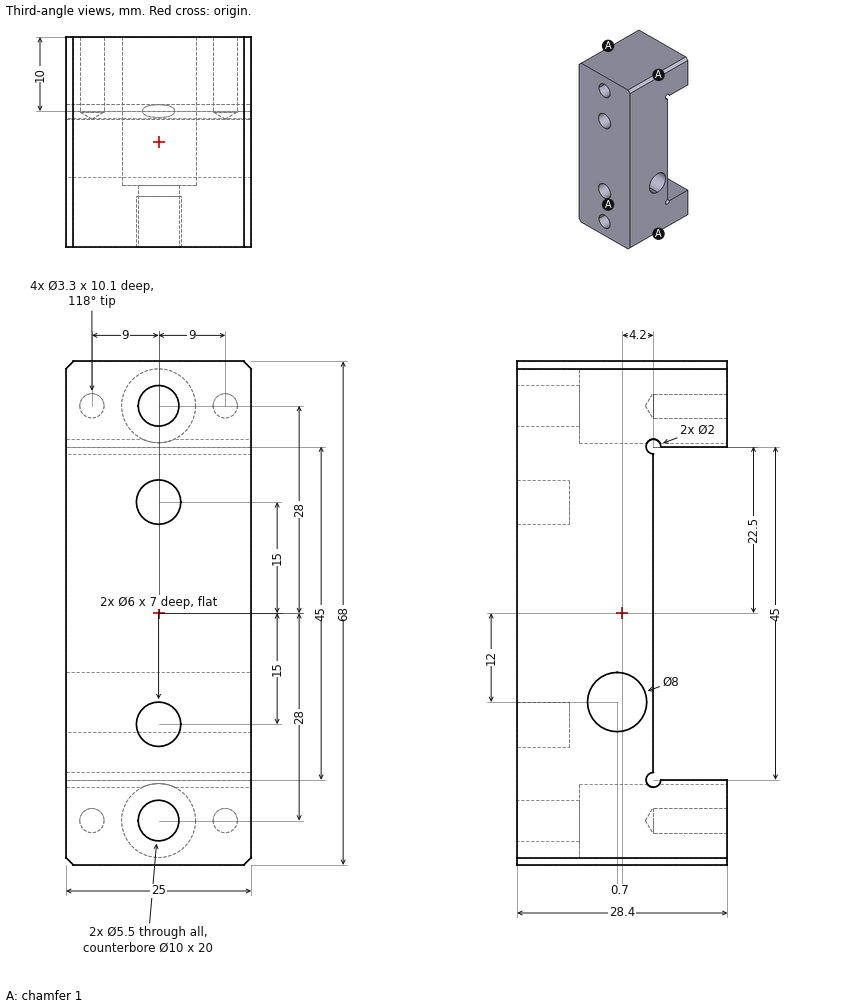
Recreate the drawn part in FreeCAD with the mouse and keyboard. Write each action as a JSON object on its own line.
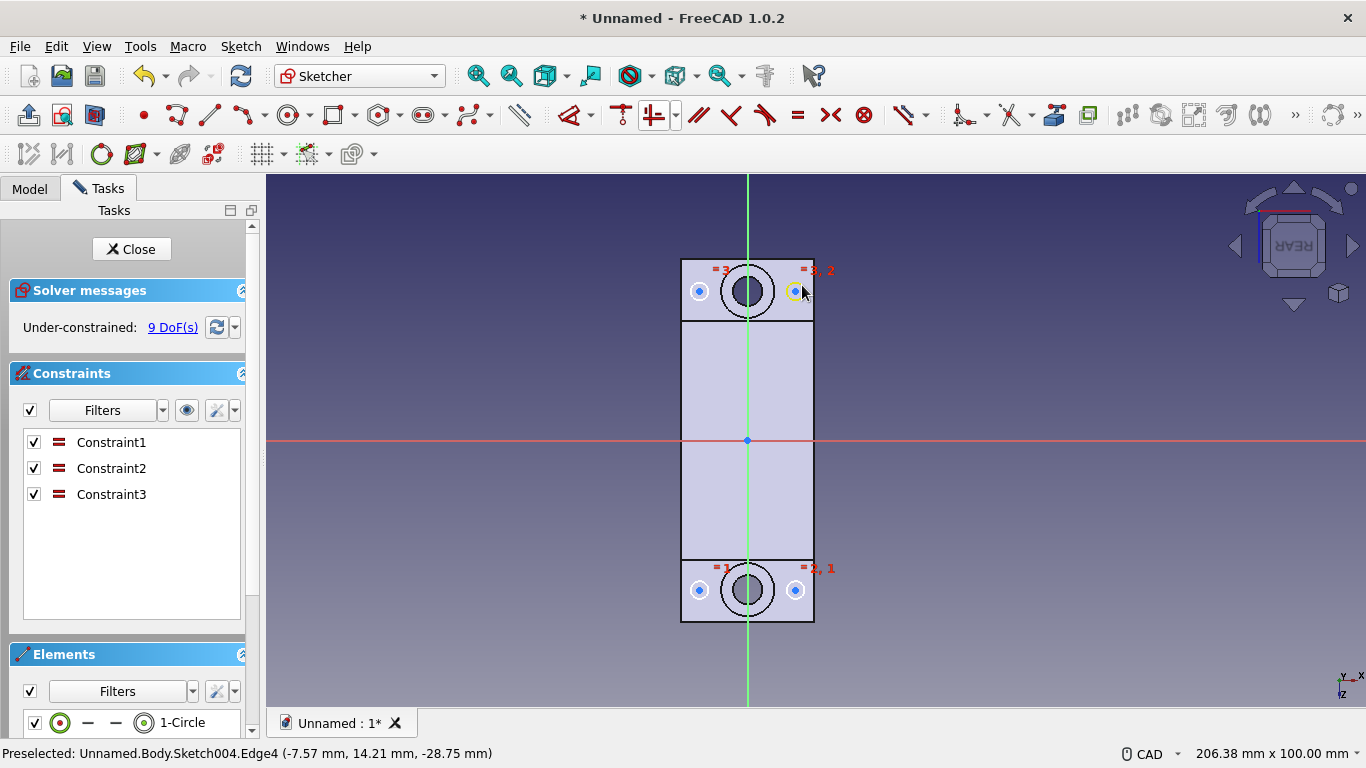
{"action": "left_click", "coordinate": [700, 590]}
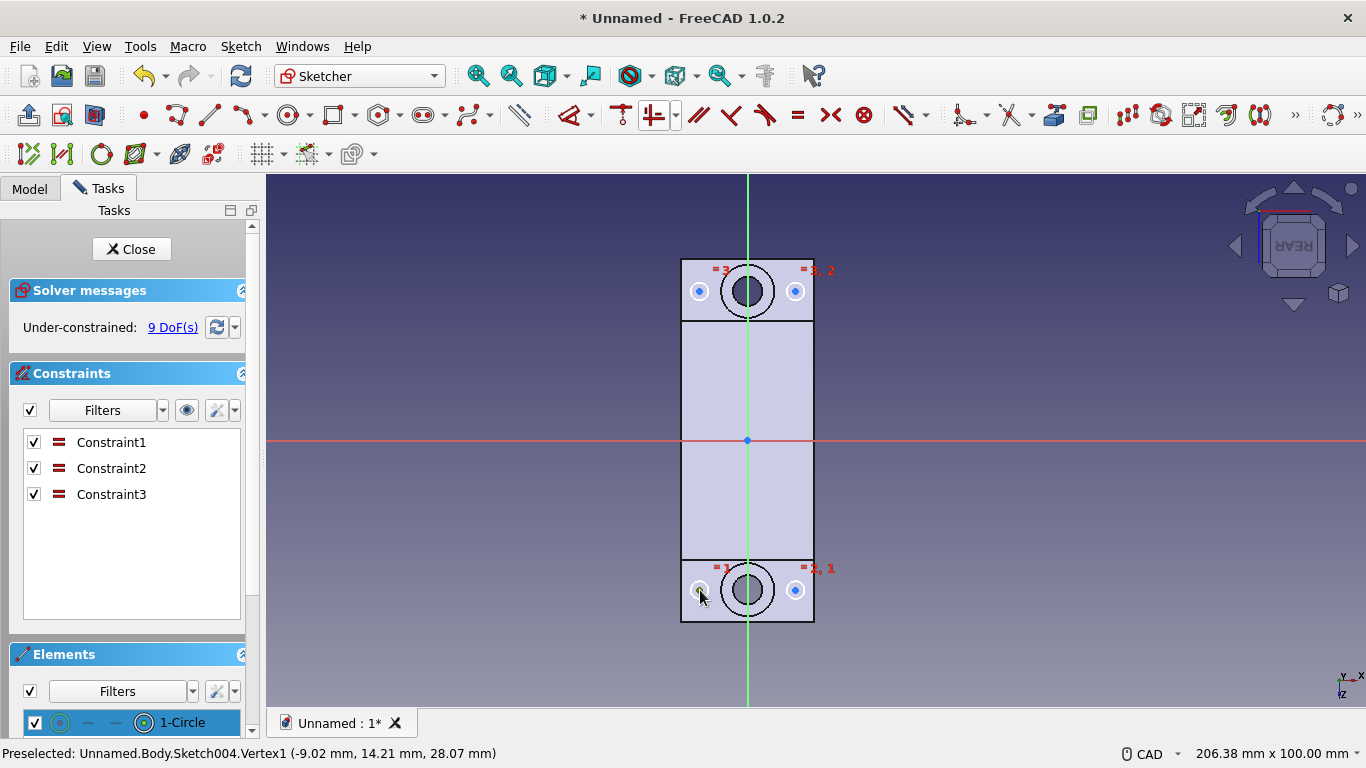
{"action": "left_click", "coordinate": [796, 590]}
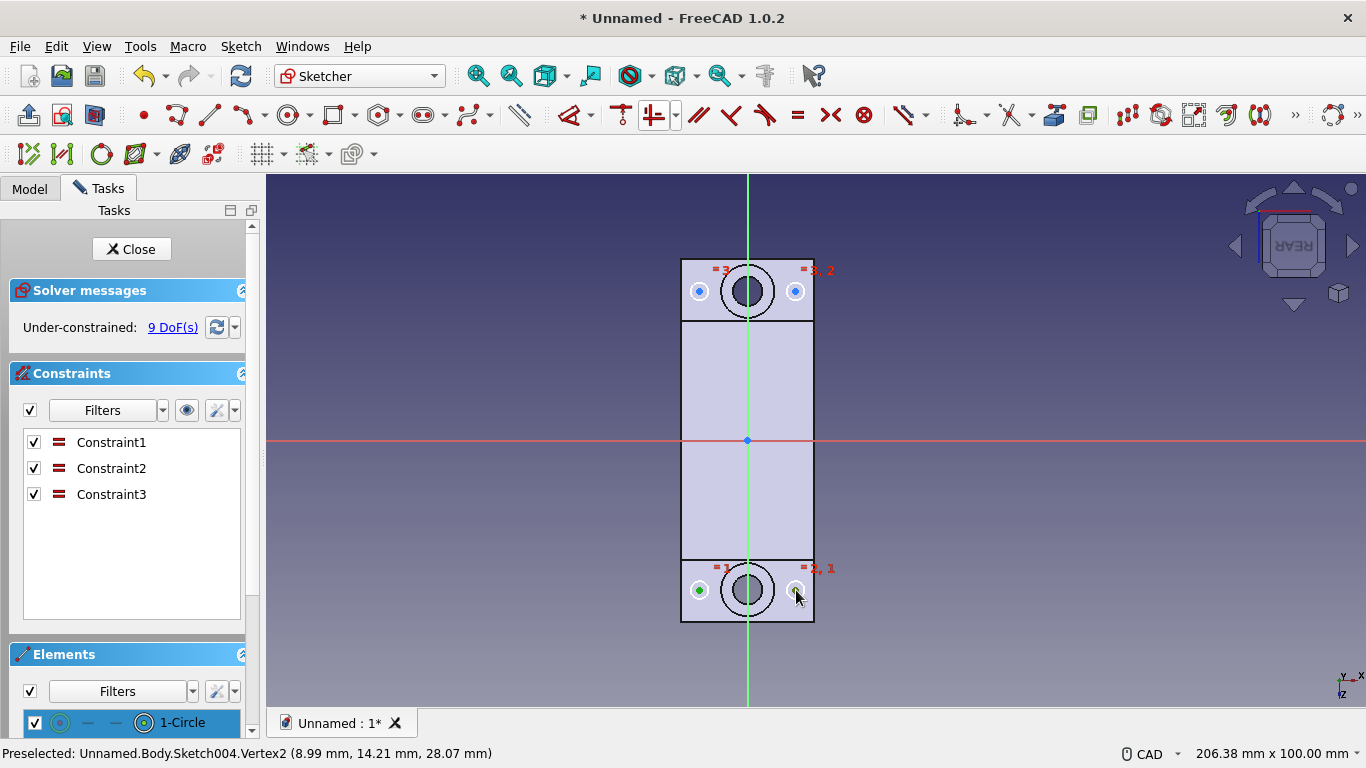
{"action": "key", "text": "h"}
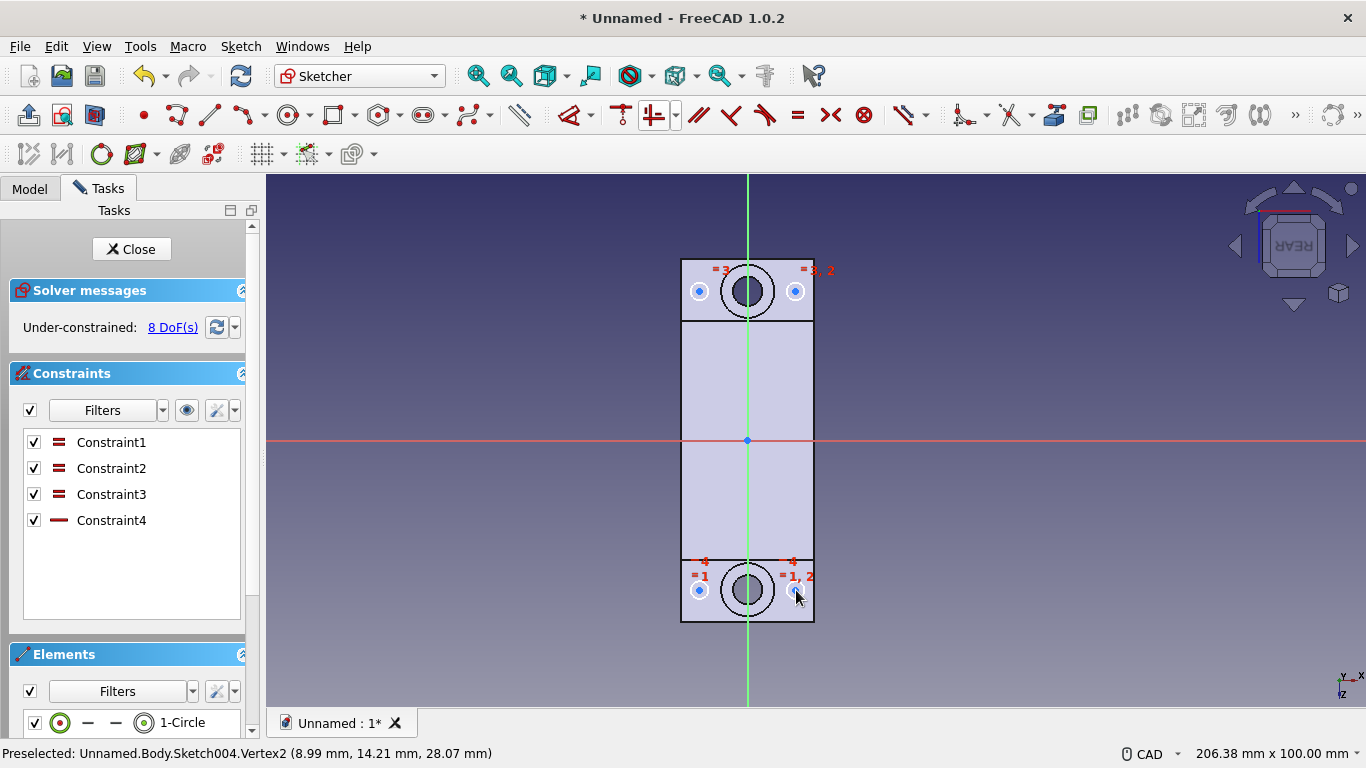
{"action": "left_click", "coordinate": [796, 590]}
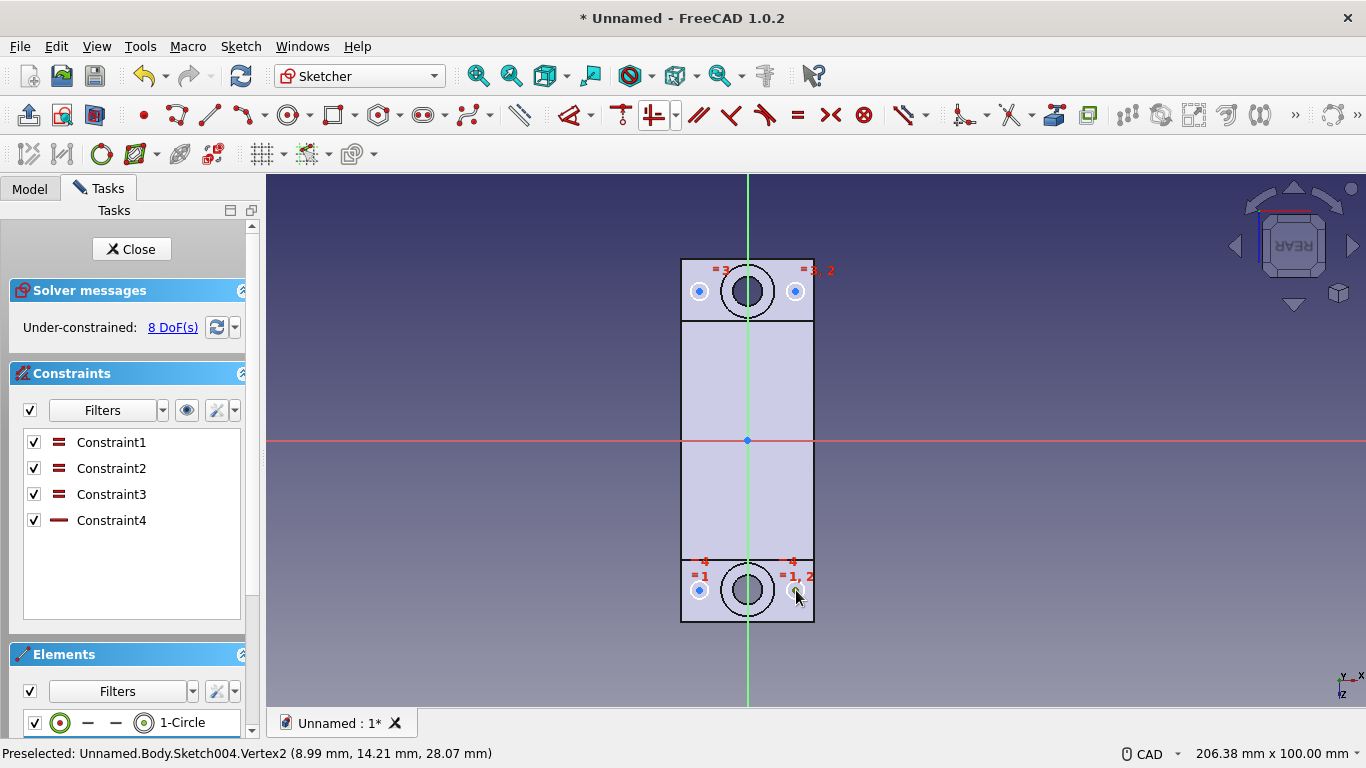
{"action": "left_click", "coordinate": [796, 292]}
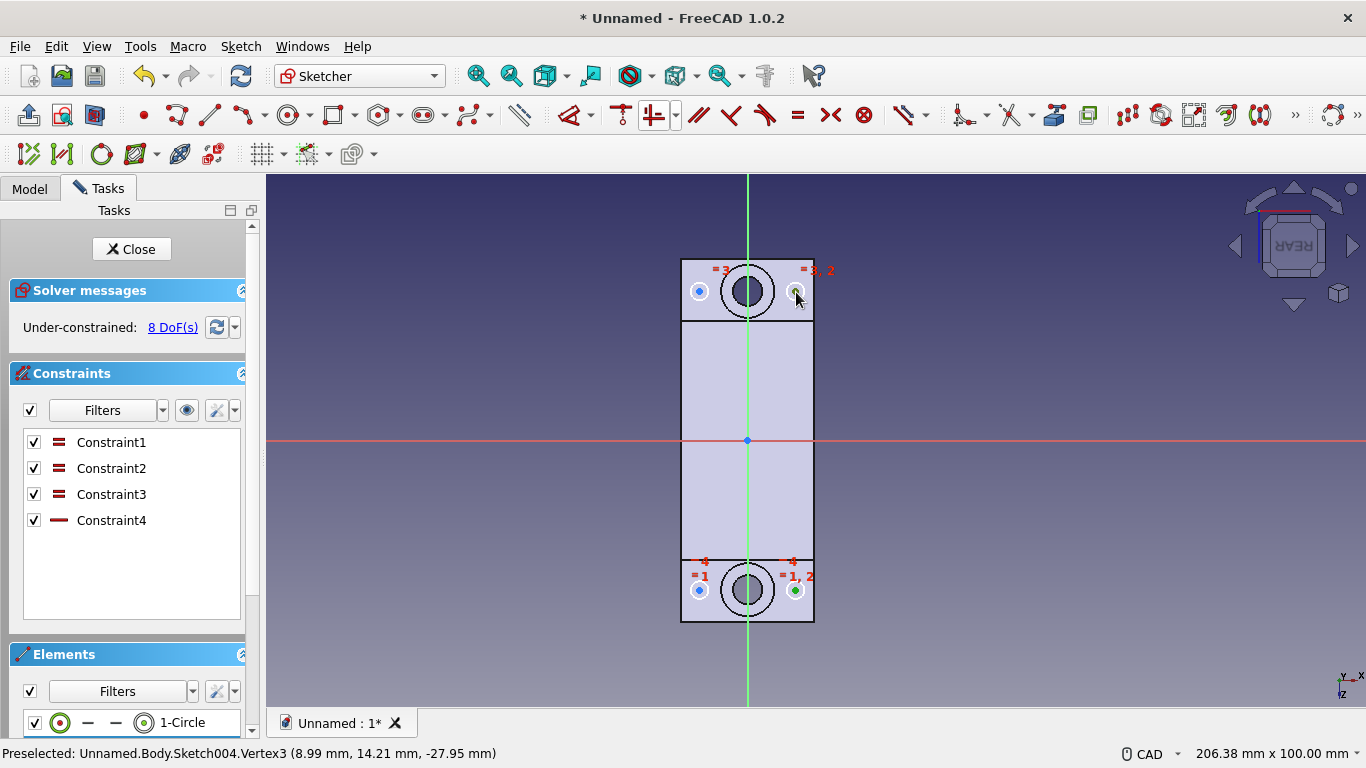
{"action": "key", "text": "v"}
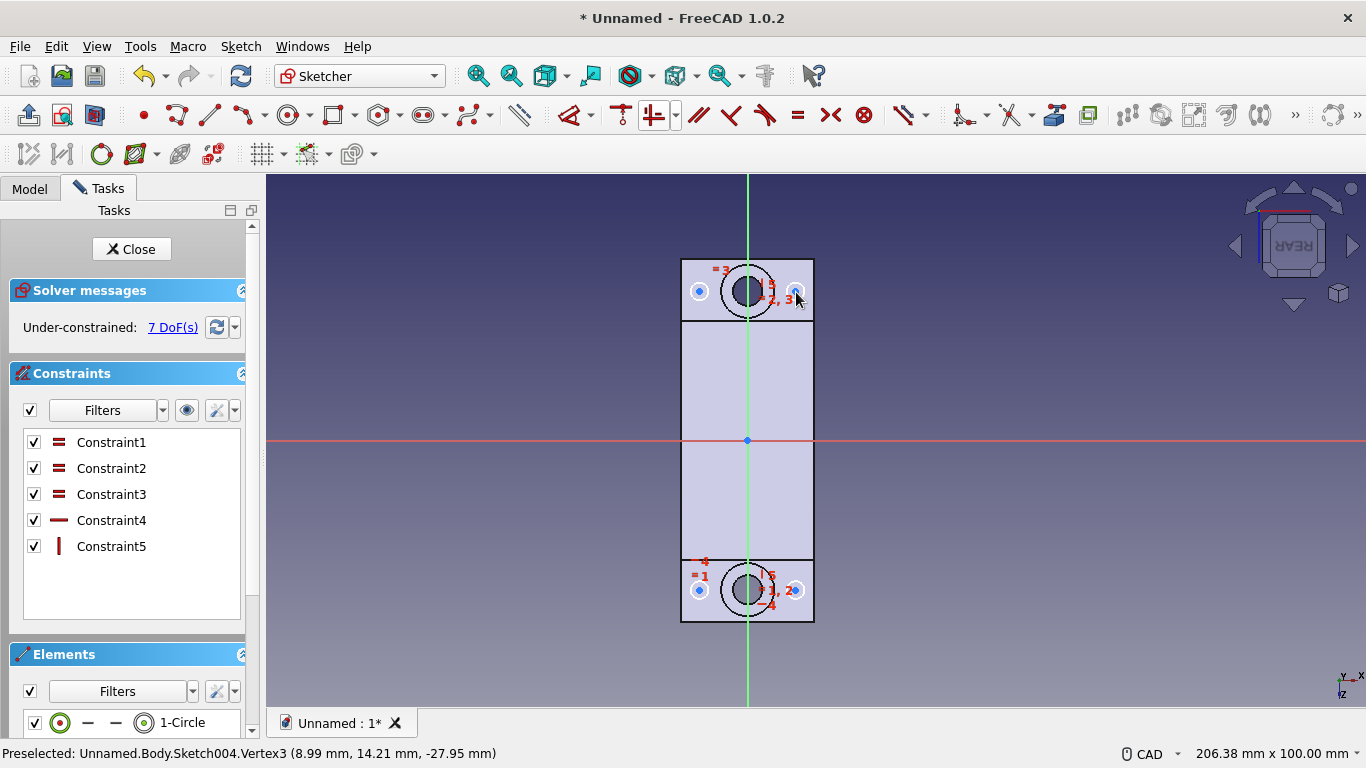
{"action": "left_click", "coordinate": [700, 590]}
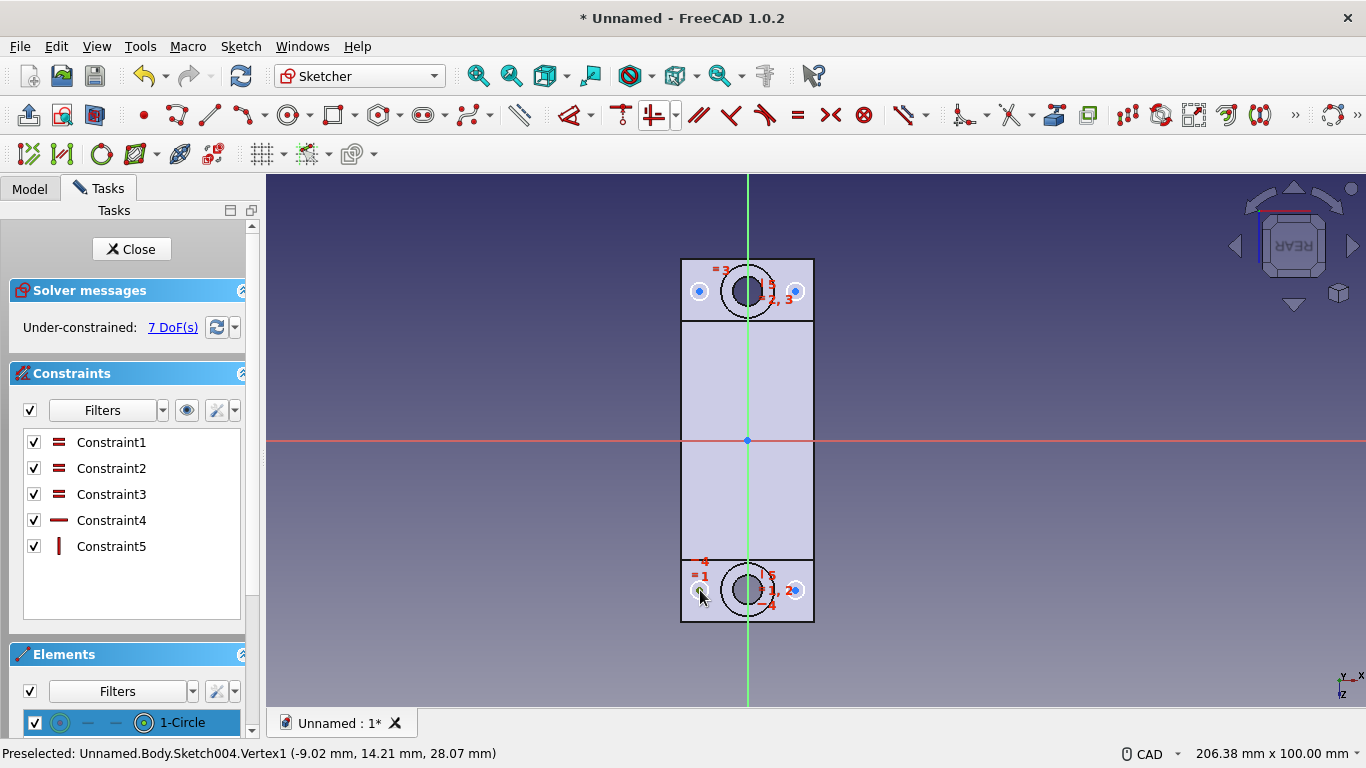
{"action": "left_click", "coordinate": [700, 292]}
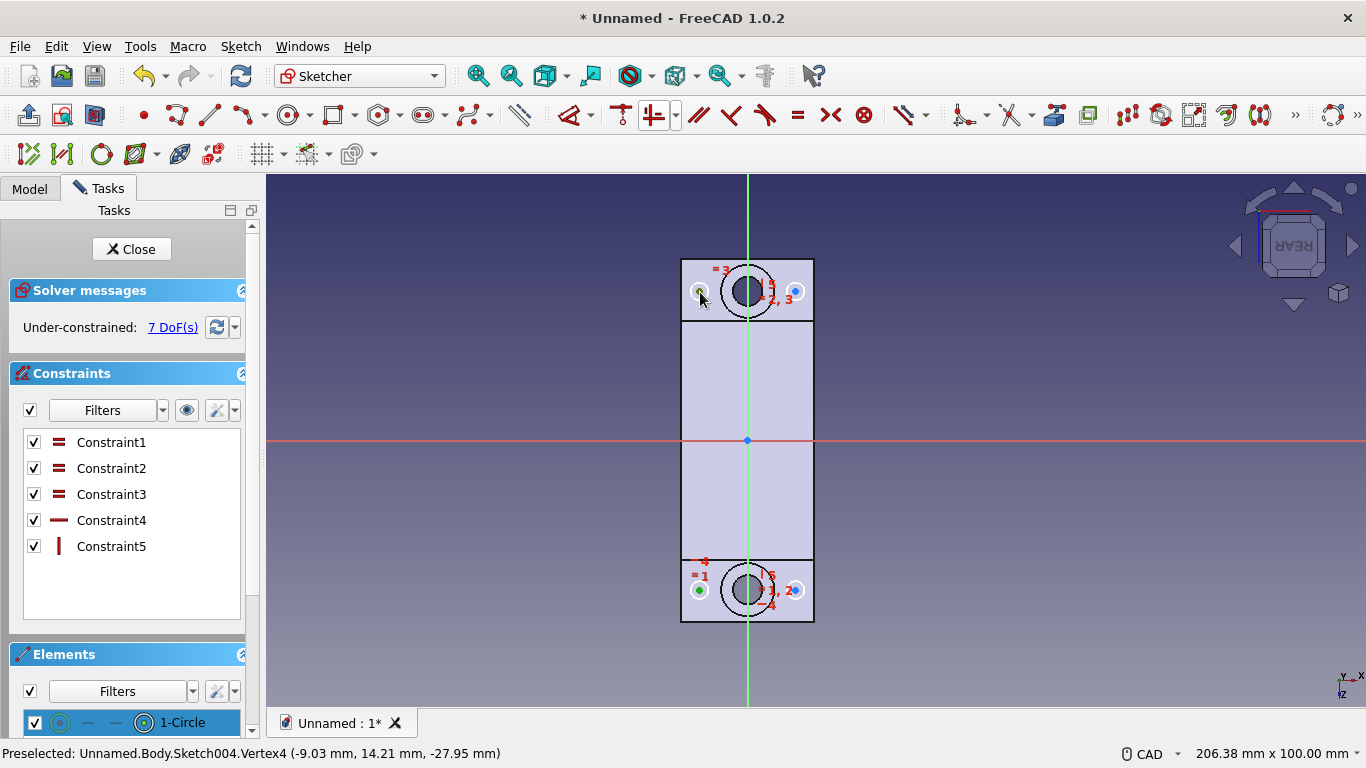
{"action": "key", "text": "v"}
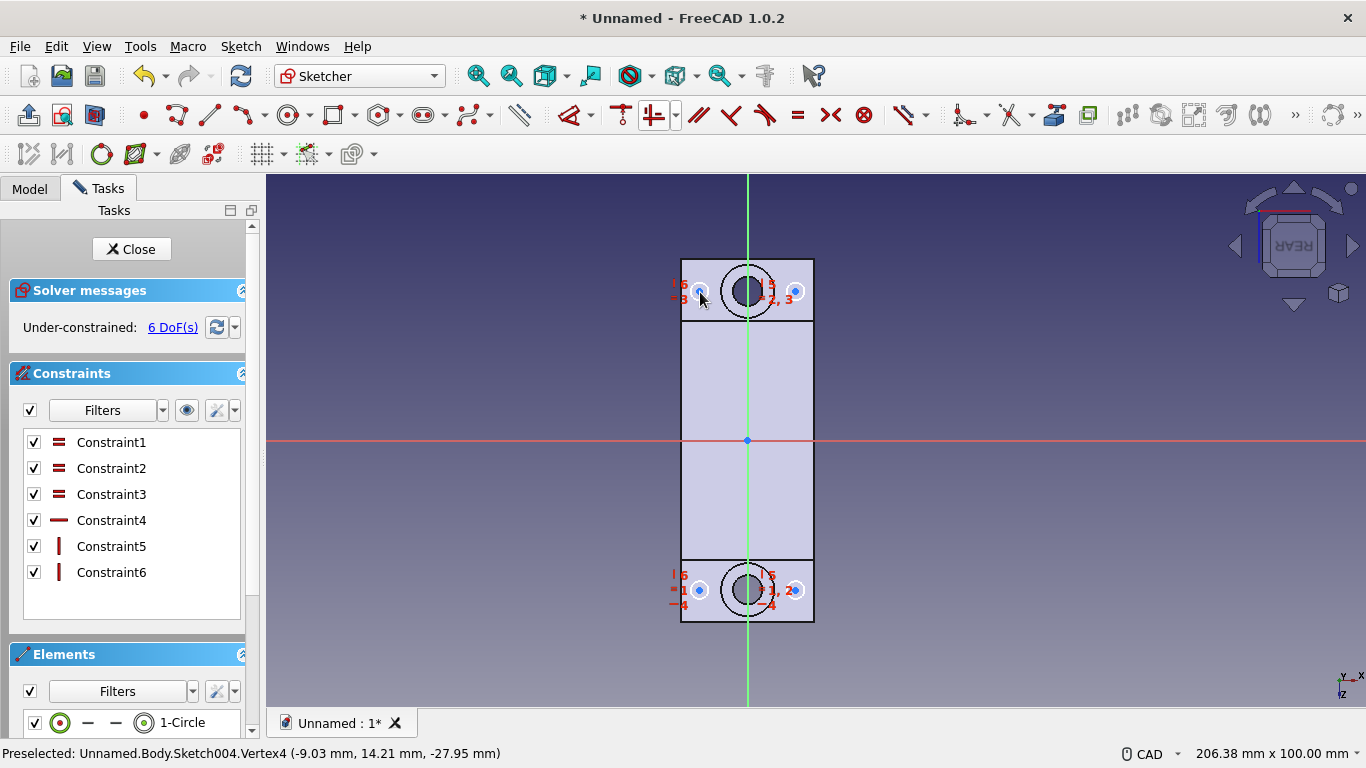
{"action": "left_click", "coordinate": [796, 292]}